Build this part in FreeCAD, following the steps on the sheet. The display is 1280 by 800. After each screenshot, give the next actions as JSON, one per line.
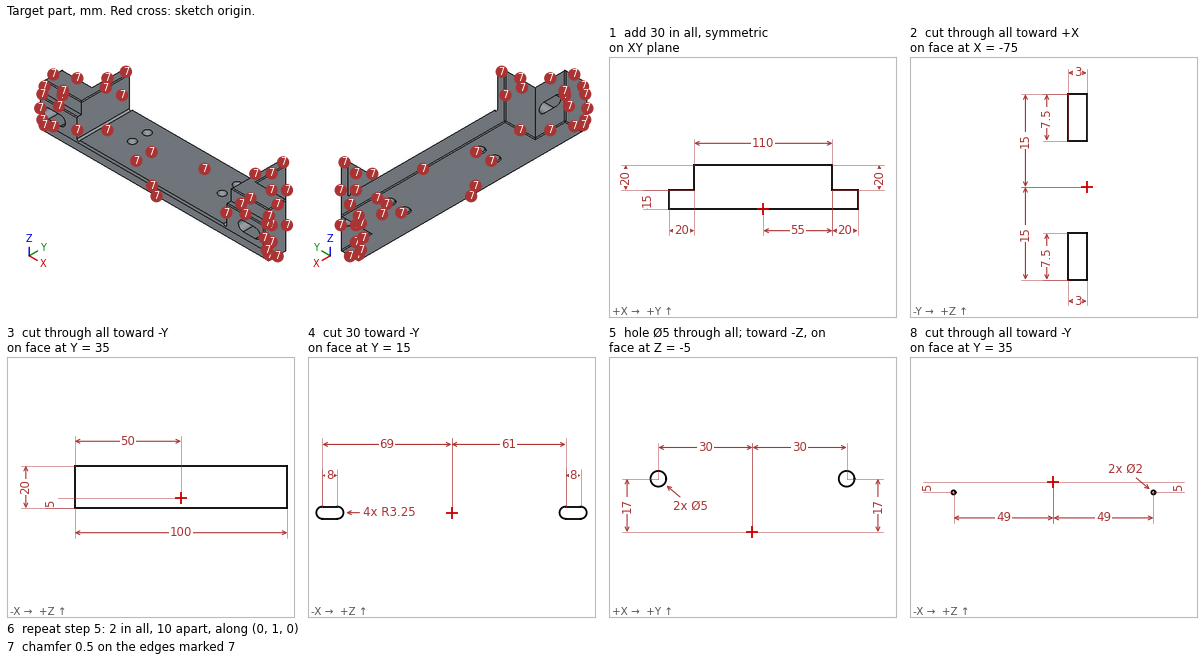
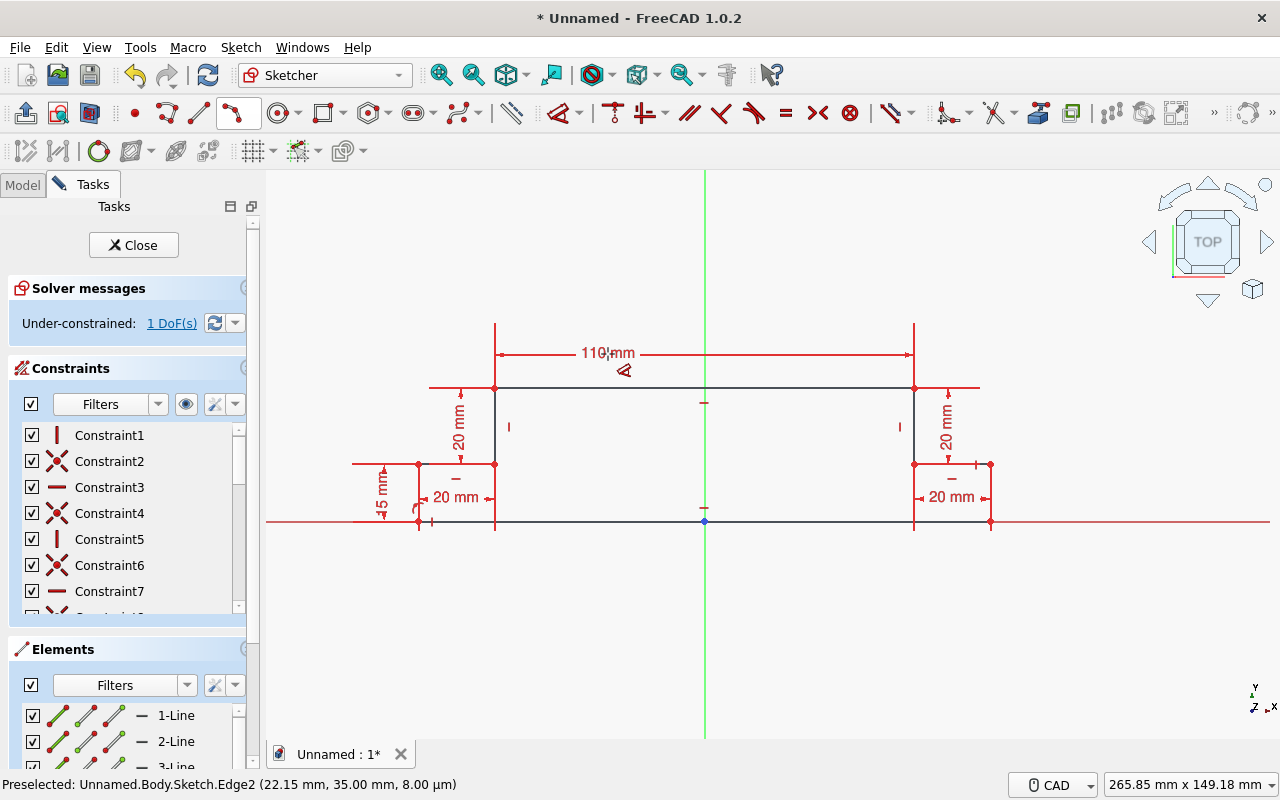
{"action": "left_click", "coordinate": [914, 464]}
{"action": "left_click", "coordinate": [809, 556]}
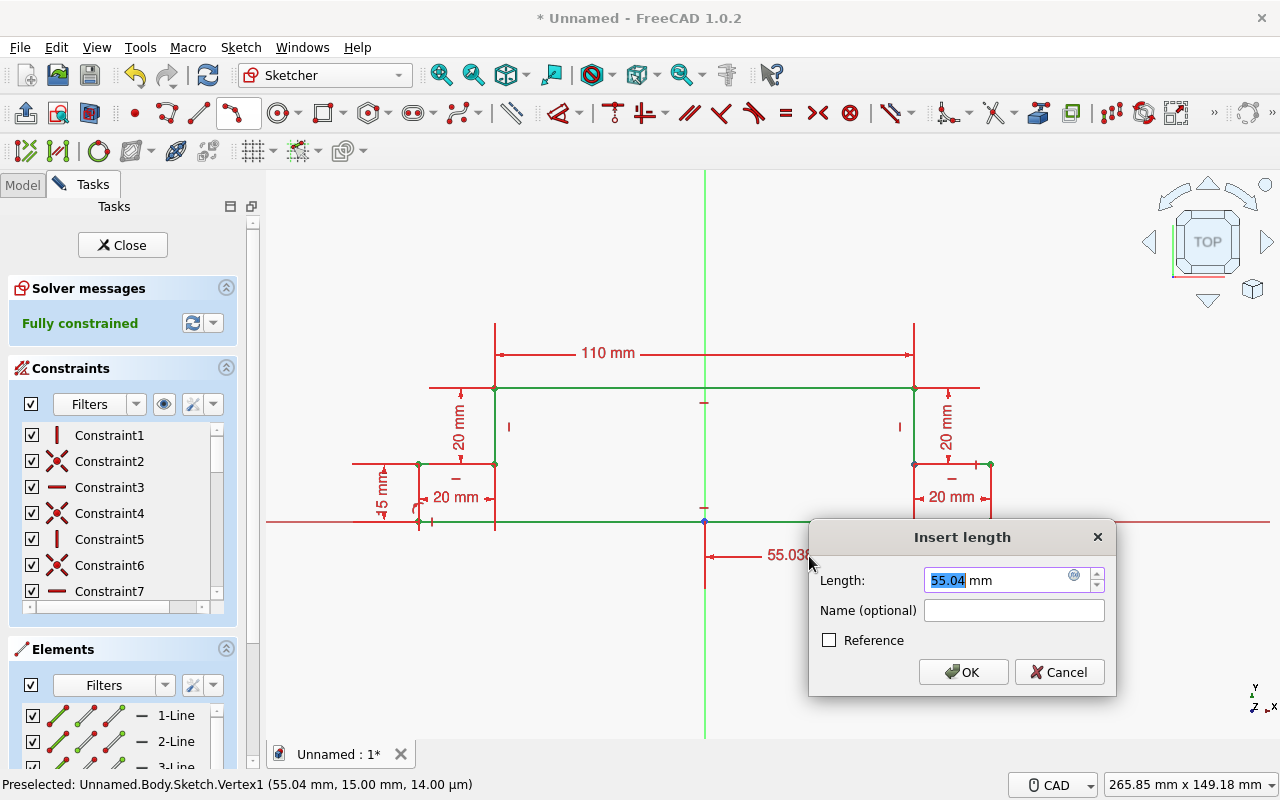
{"action": "type", "text": "55"}
{"action": "key", "text": "Return"}
{"action": "key", "text": "Escape"}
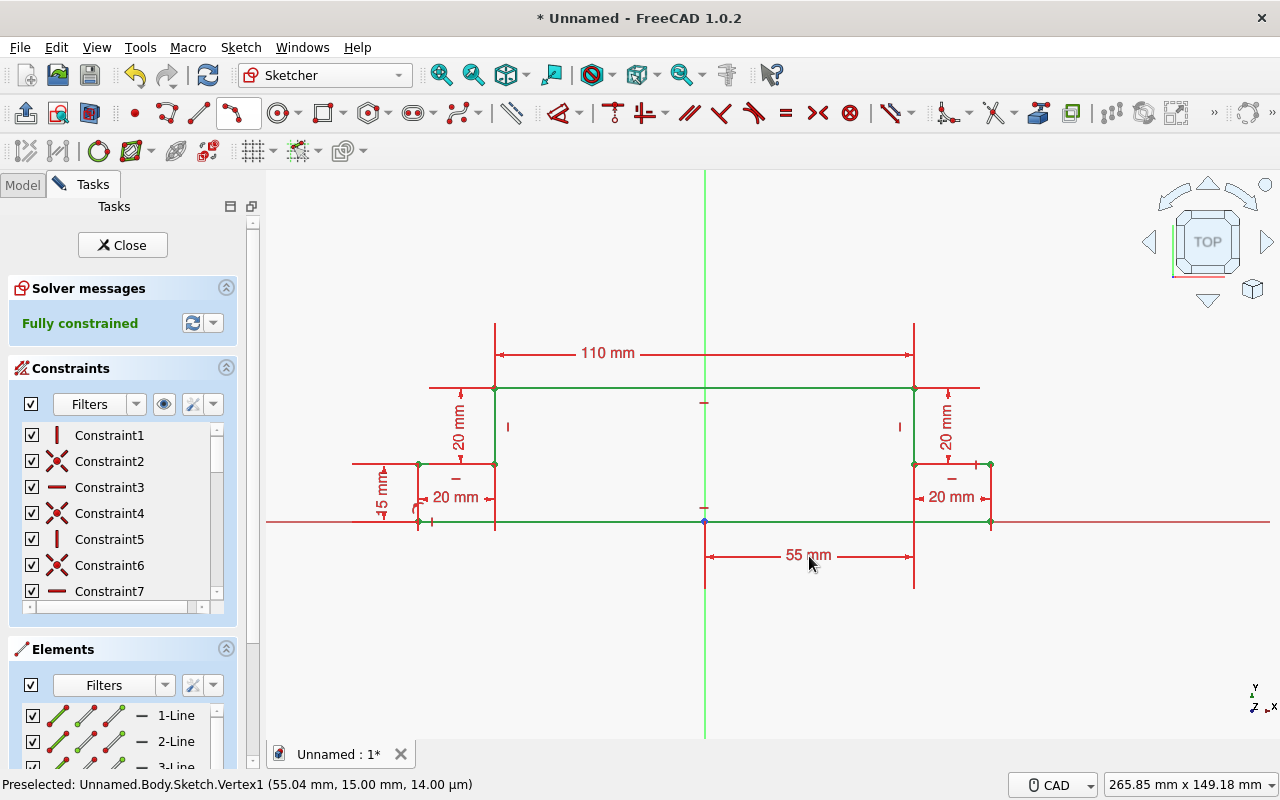
{"action": "left_click", "coordinate": [123, 245]}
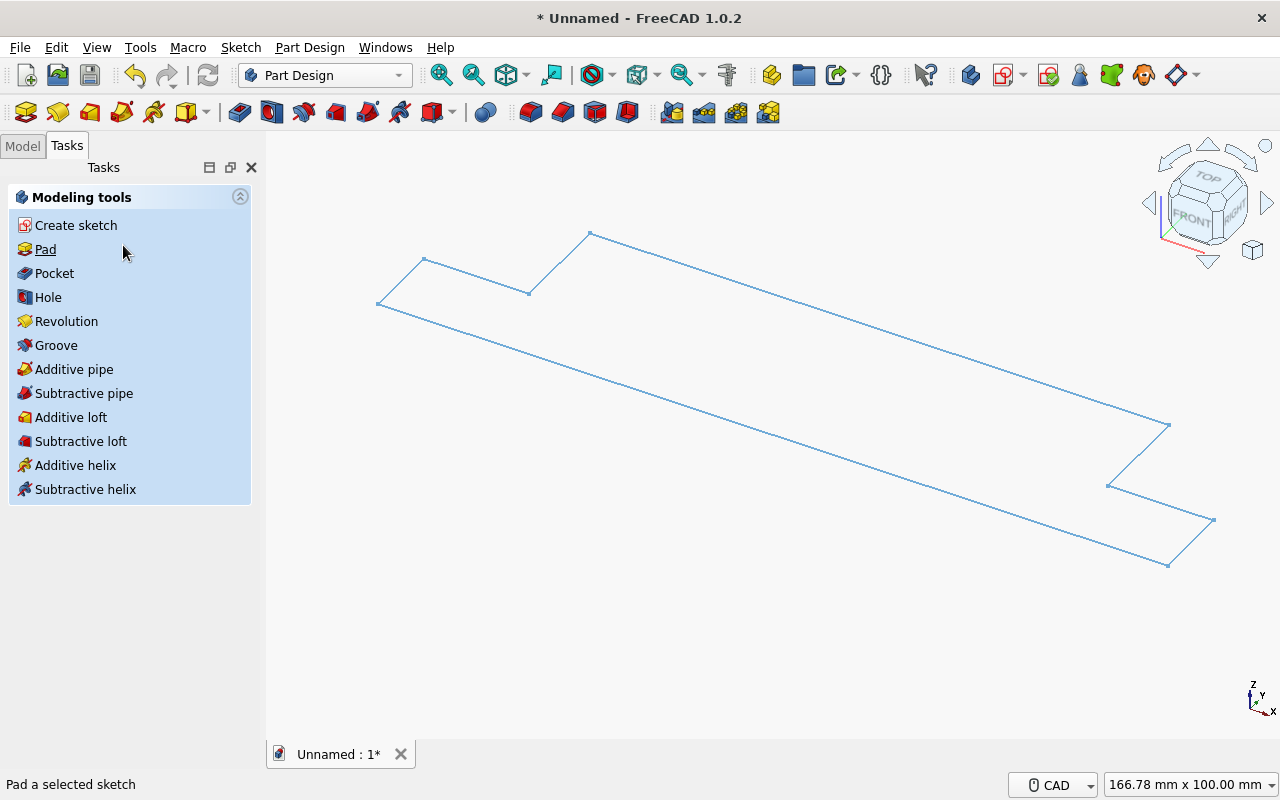
{"action": "left_click", "coordinate": [26, 112]}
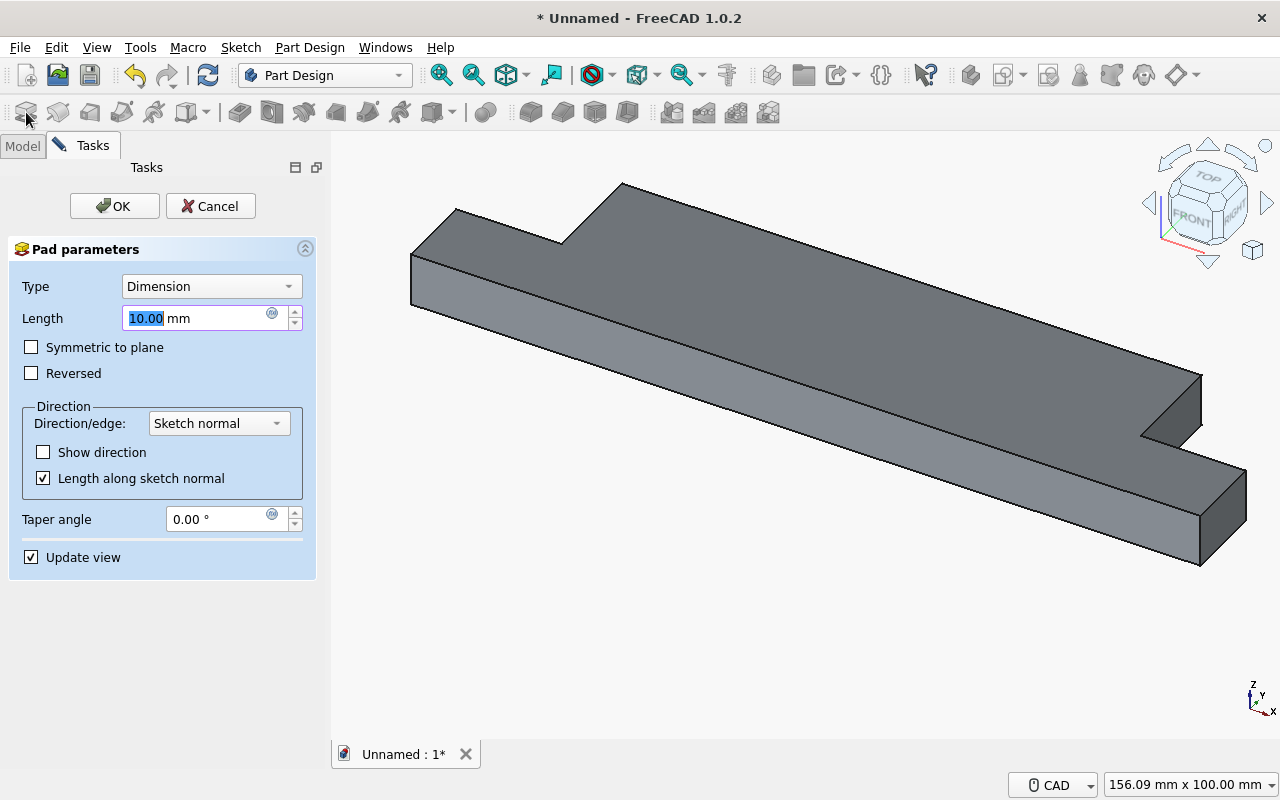
{"action": "type", "text": "30"}
{"action": "key", "text": "Tab"}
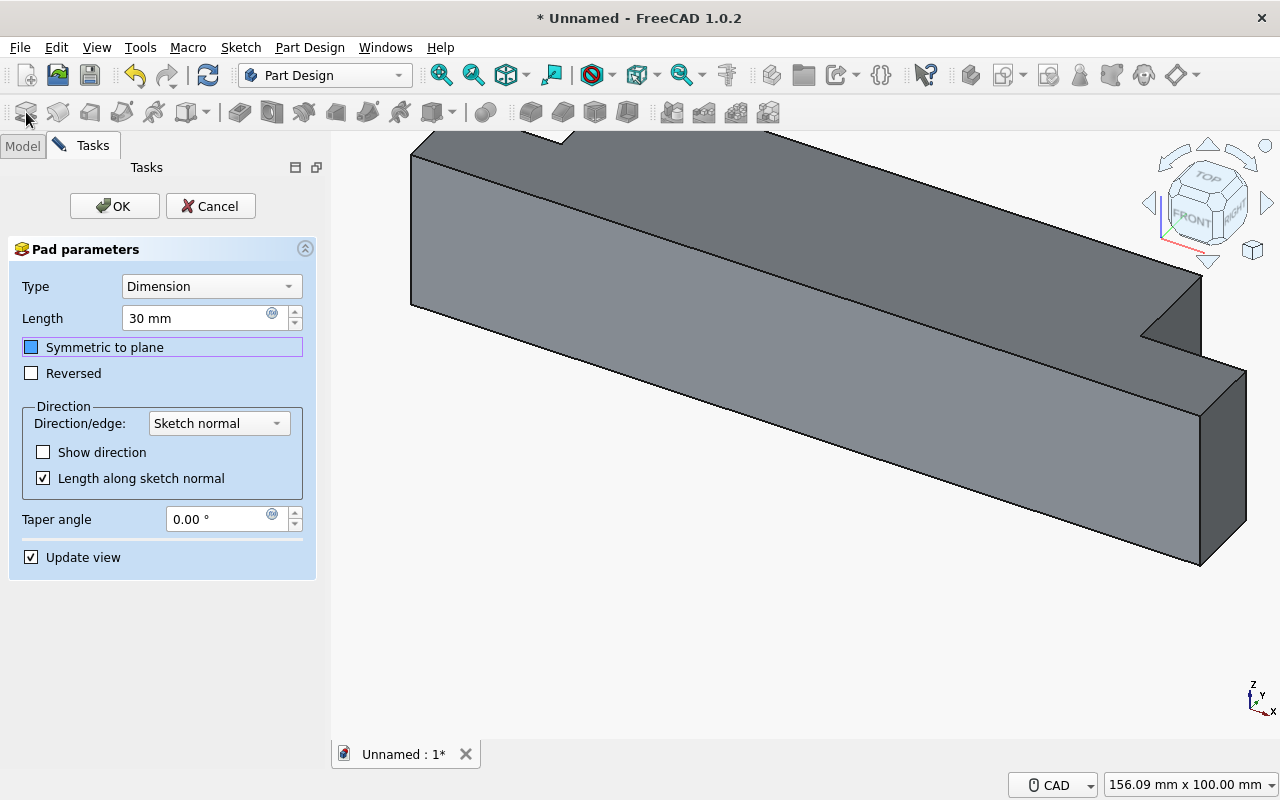
{"action": "left_click", "coordinate": [30, 347]}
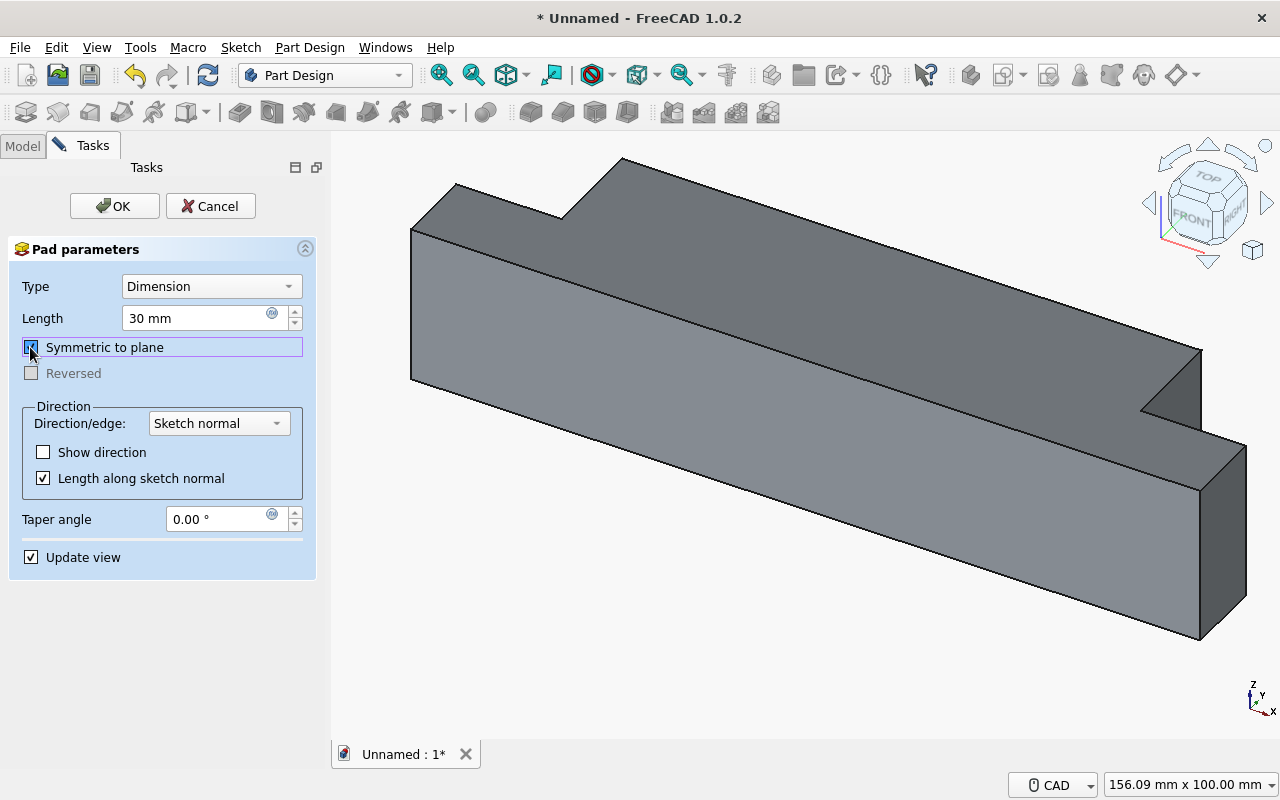
{"action": "left_click", "coordinate": [115, 206]}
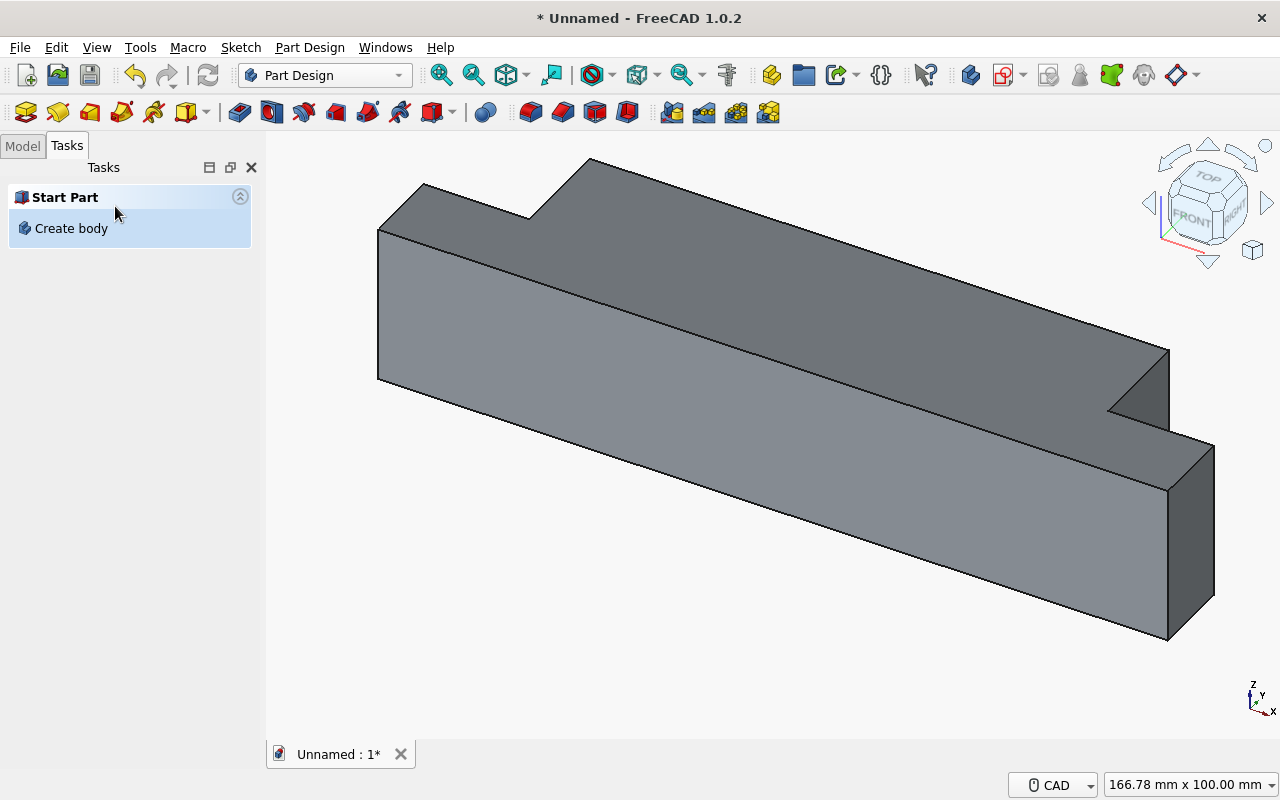
{"action": "key", "text": "v f"}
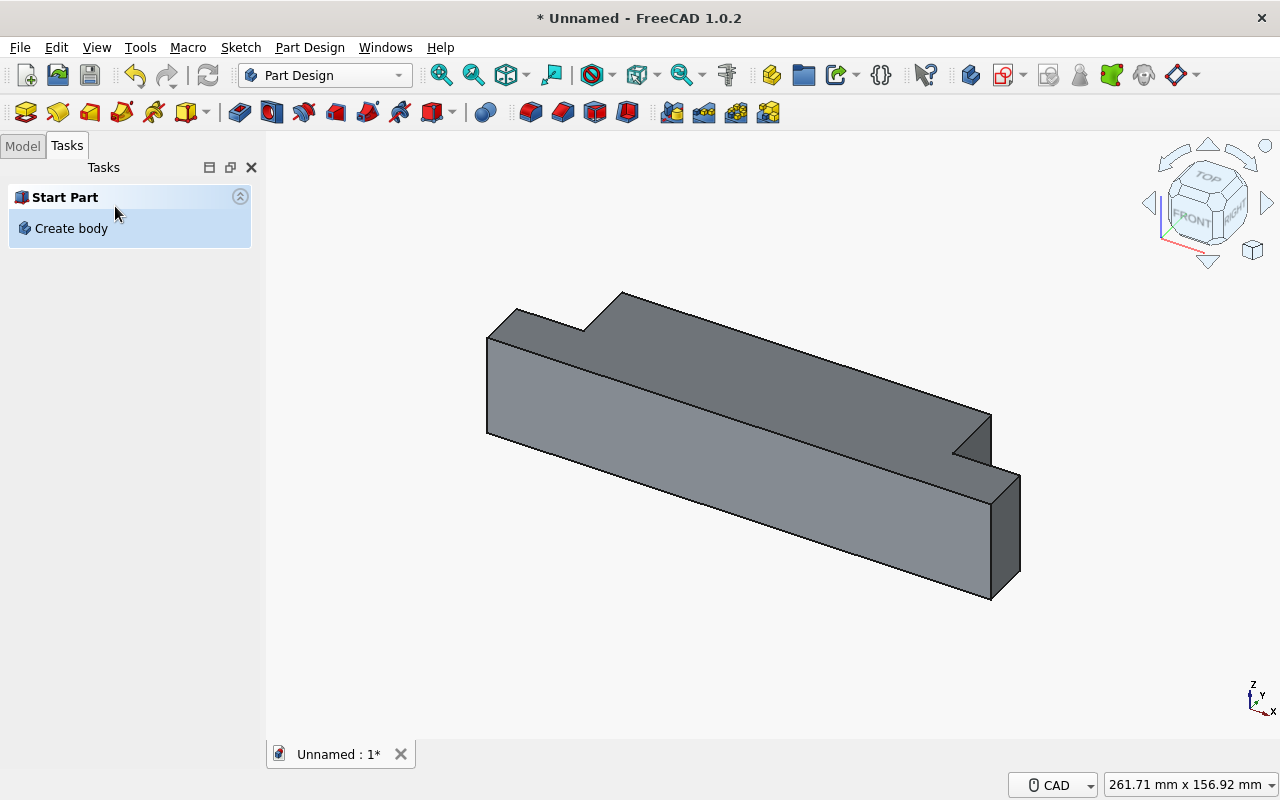
{"action": "key", "text": "6"}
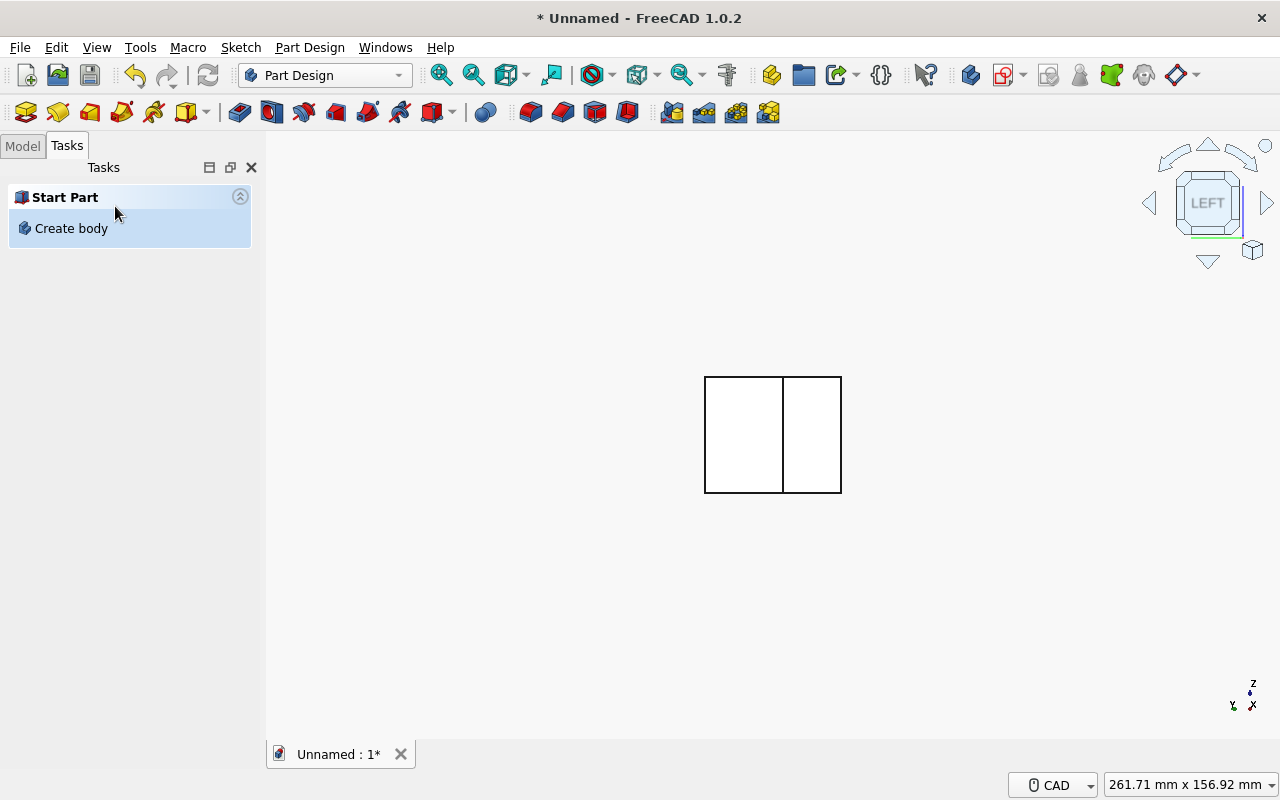
{"action": "key", "text": "v f"}